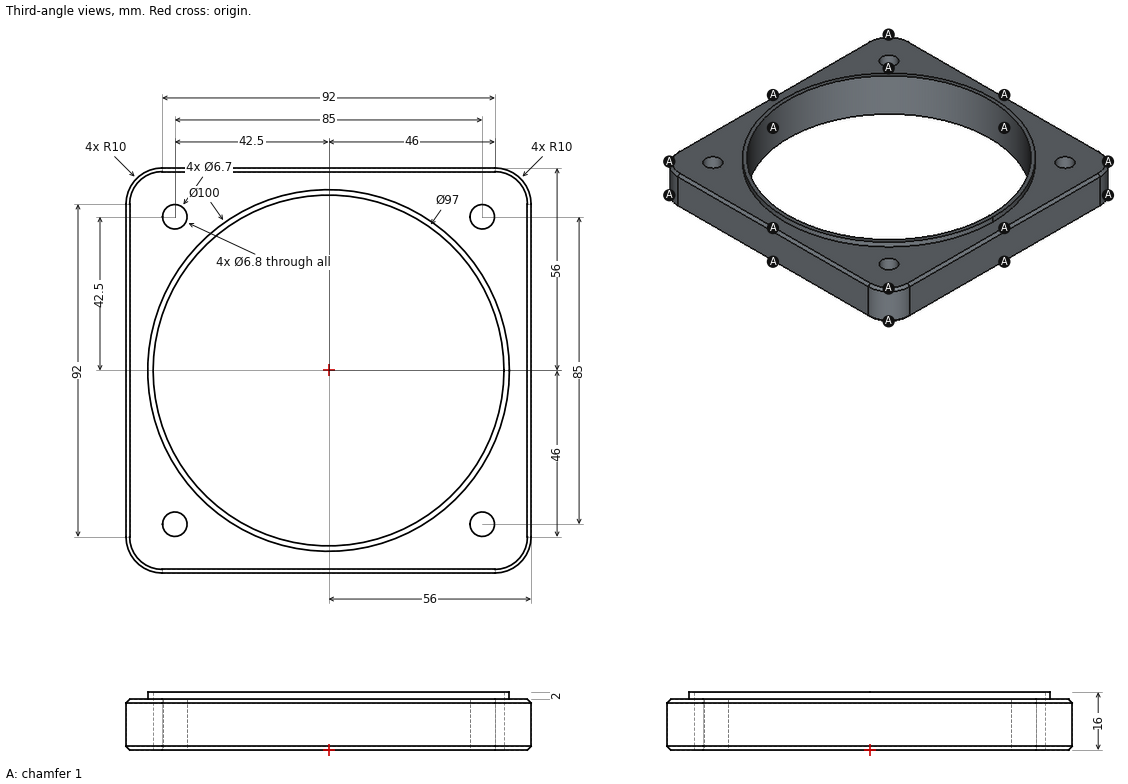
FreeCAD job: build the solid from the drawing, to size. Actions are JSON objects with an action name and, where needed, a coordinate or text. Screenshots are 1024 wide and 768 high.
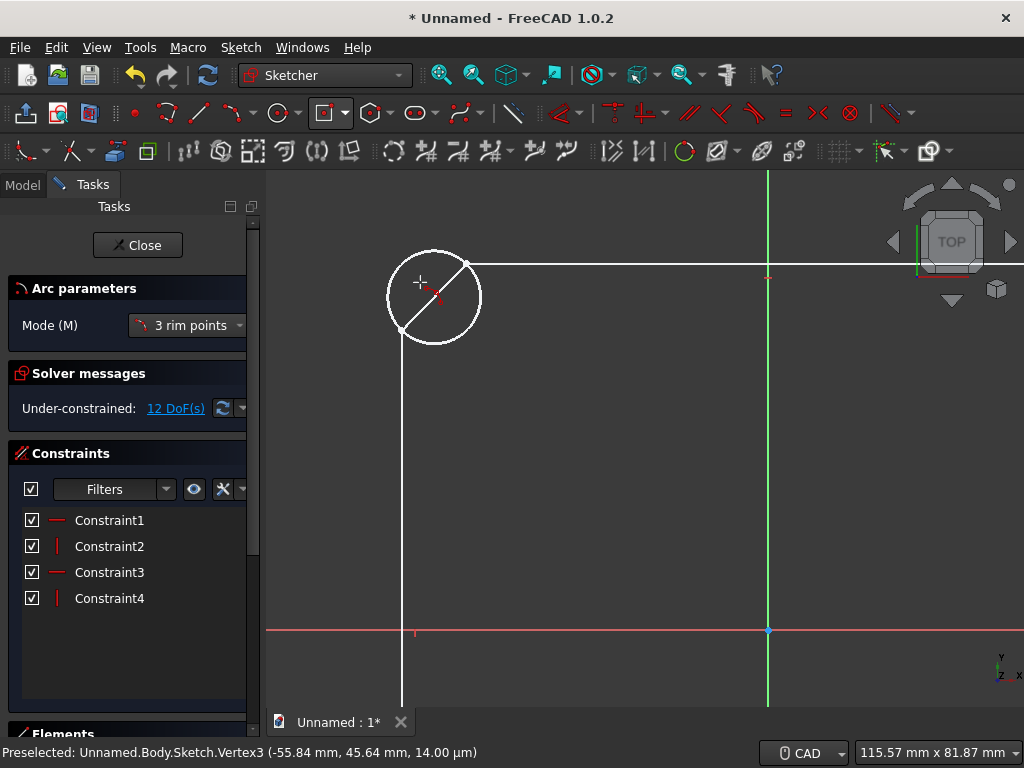
{"action": "left_click", "coordinate": [420, 282]}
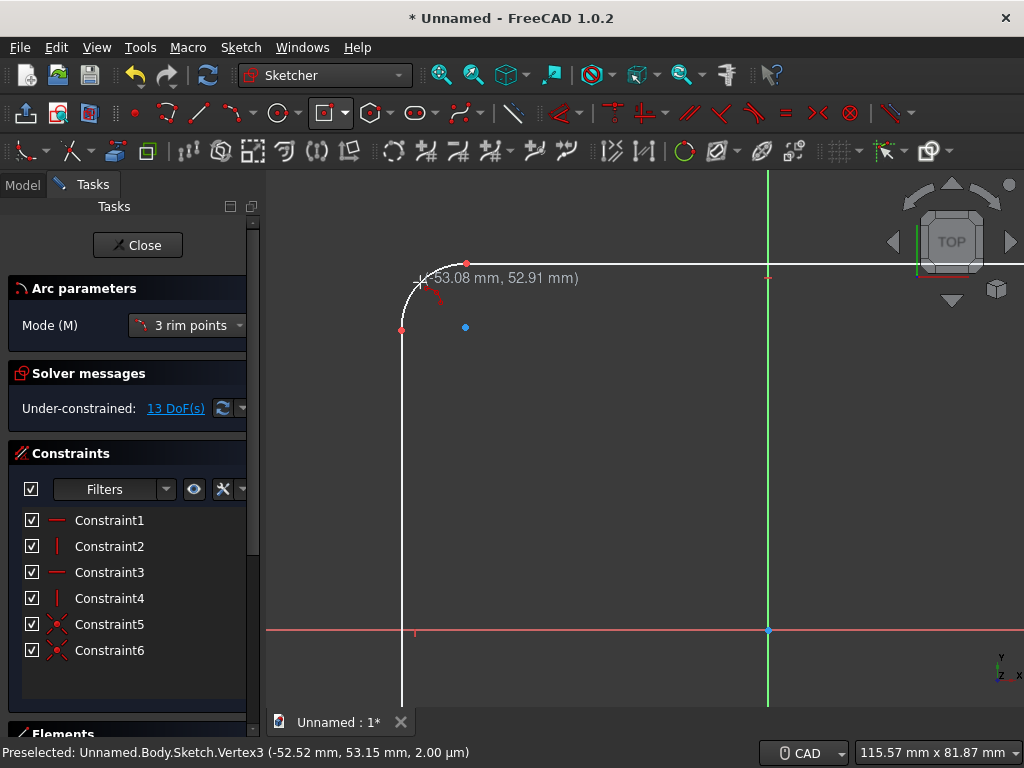
{"action": "scroll", "coordinate": [420, 282], "scroll_direction": "down", "scroll_amount": 4}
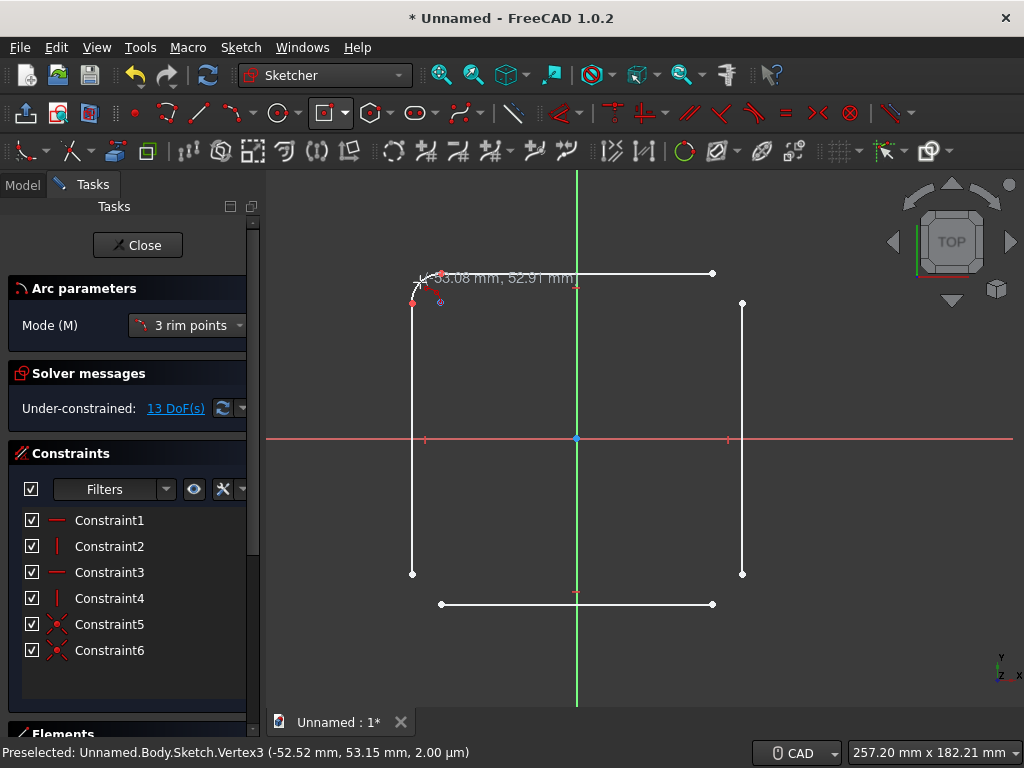
{"action": "left_click", "coordinate": [412, 575]}
{"action": "left_click", "coordinate": [441, 605]}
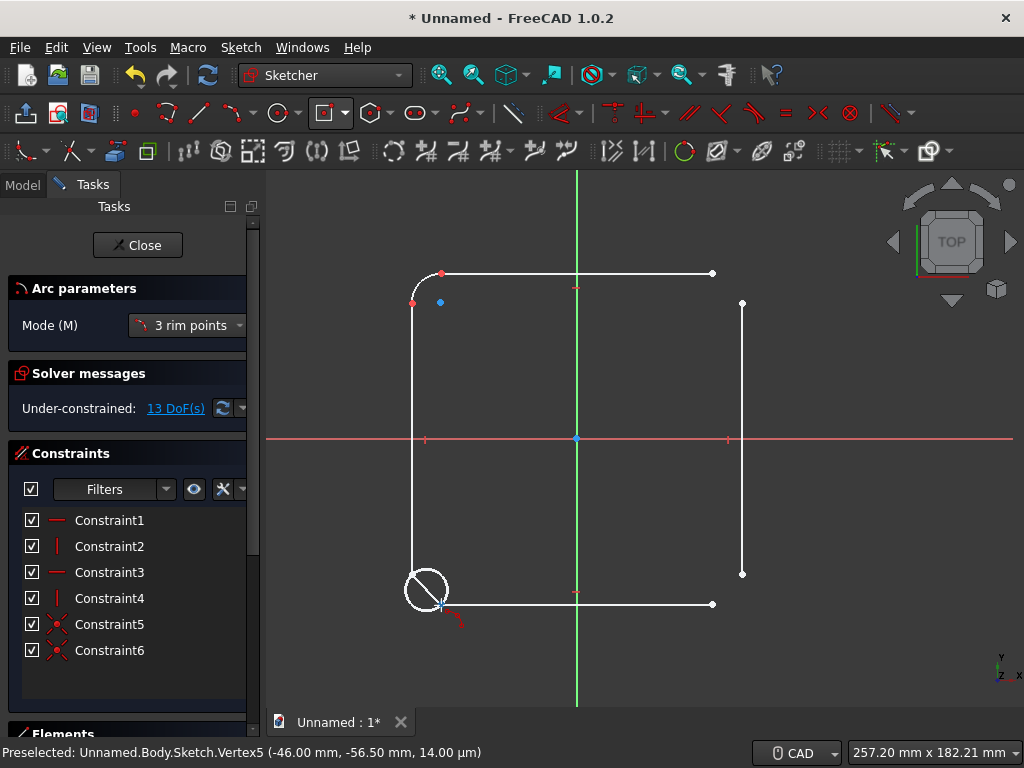
{"action": "scroll", "coordinate": [420, 595], "scroll_direction": "up", "scroll_amount": 4}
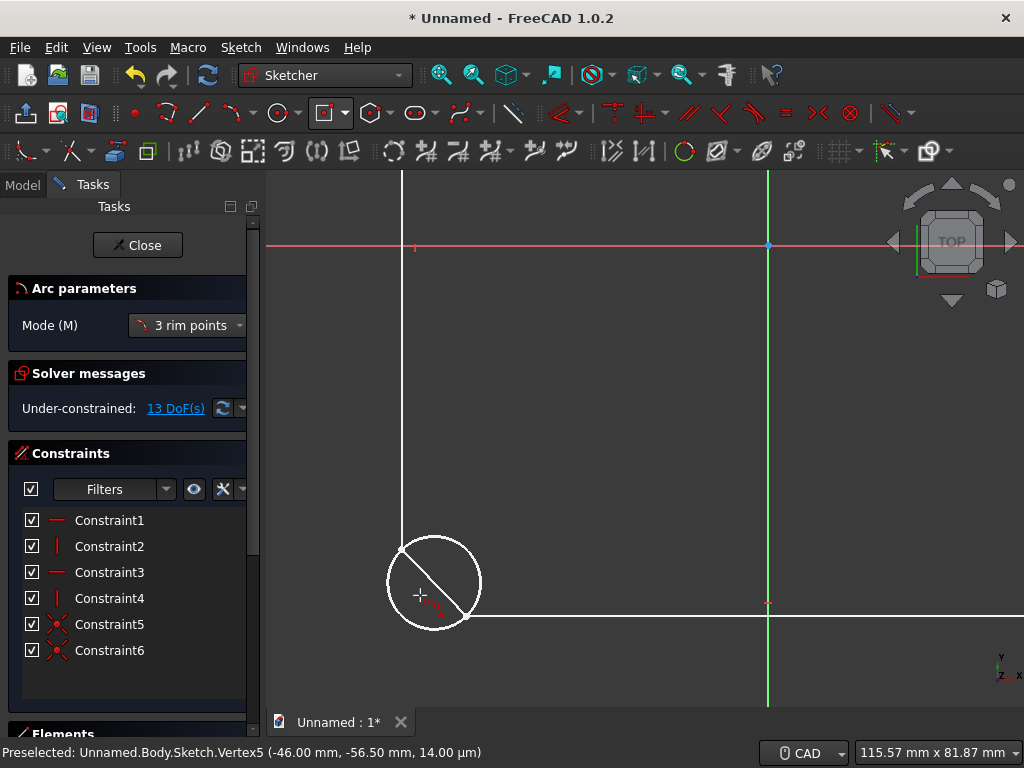
{"action": "left_click", "coordinate": [420, 594]}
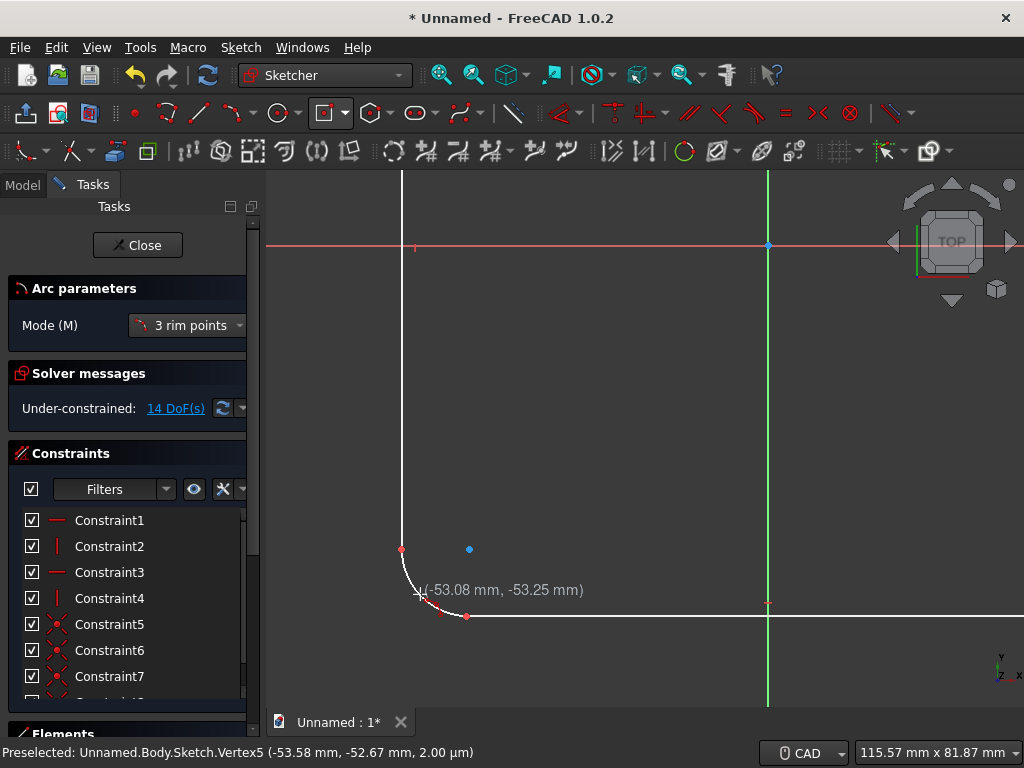
{"action": "scroll", "coordinate": [420, 596], "scroll_direction": "down", "scroll_amount": 4}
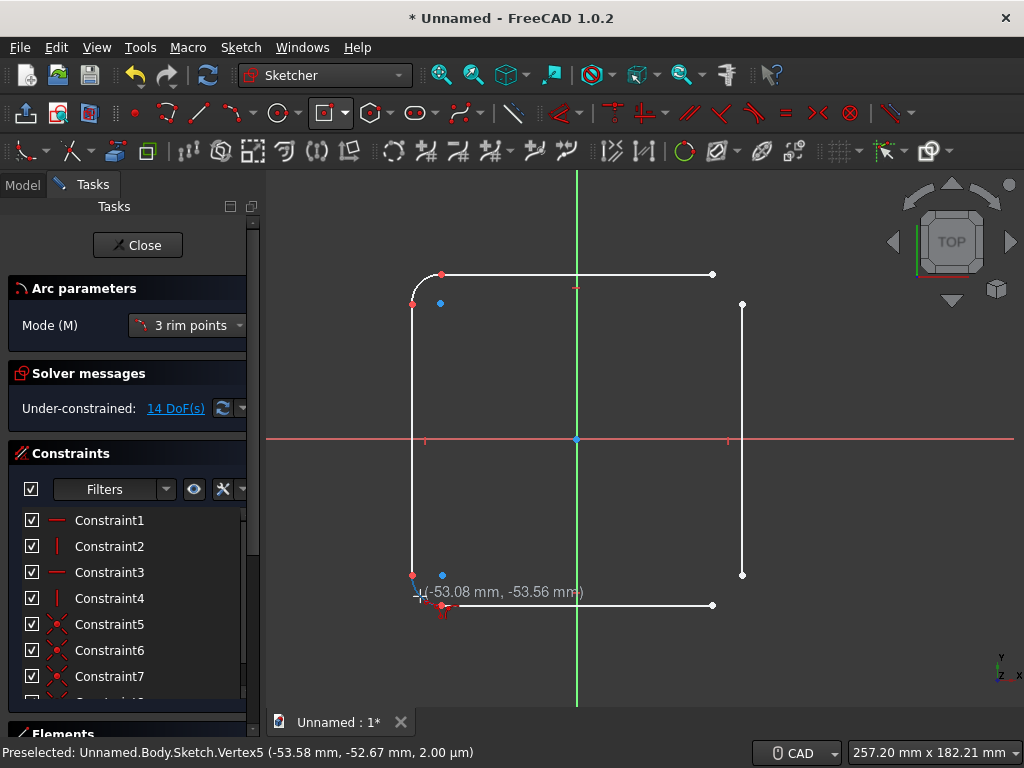
{"action": "left_click", "coordinate": [712, 606]}
{"action": "left_click", "coordinate": [742, 576]}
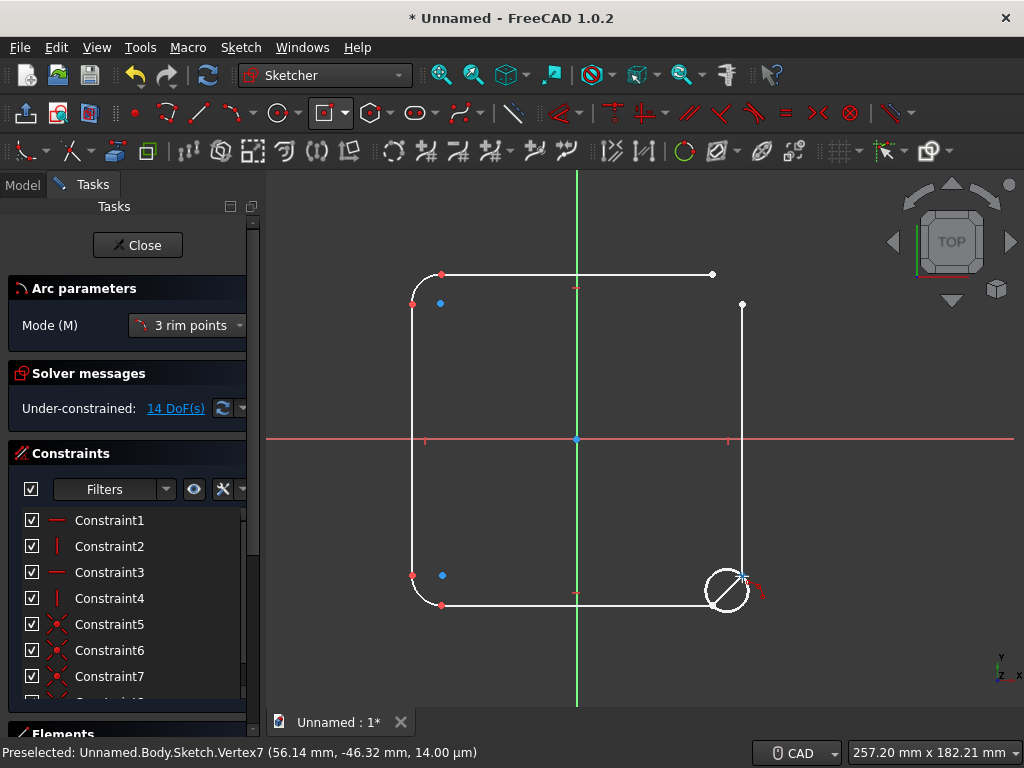
{"action": "scroll", "coordinate": [733, 595], "scroll_direction": "up", "scroll_amount": 4}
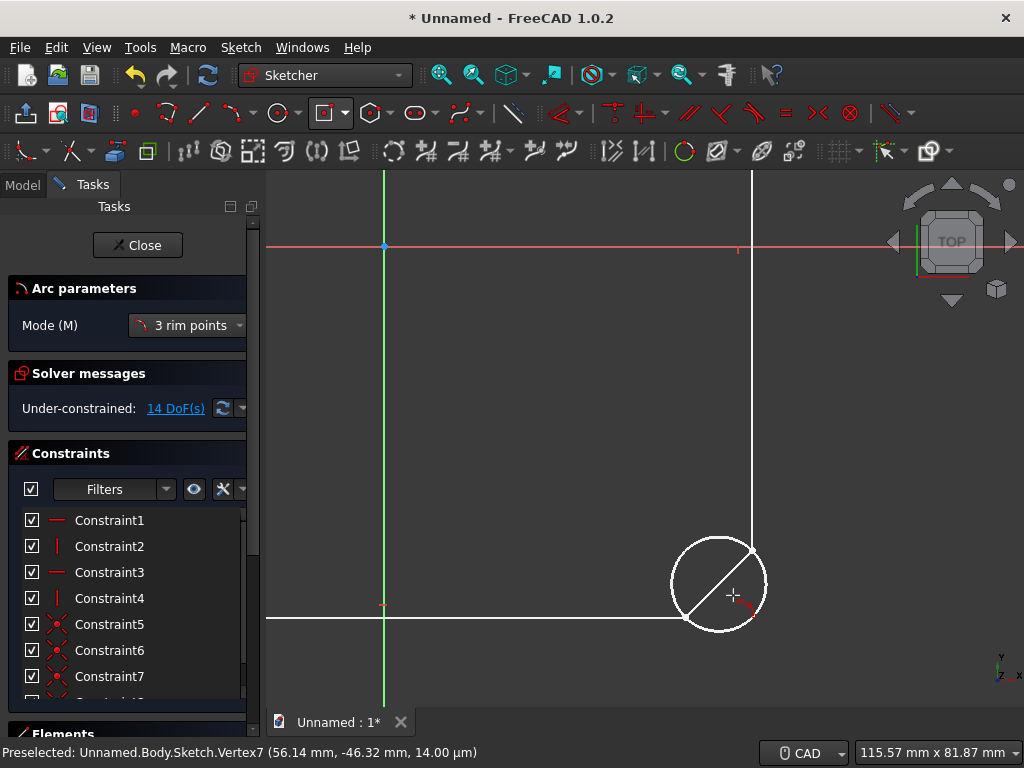
{"action": "left_click", "coordinate": [732, 595]}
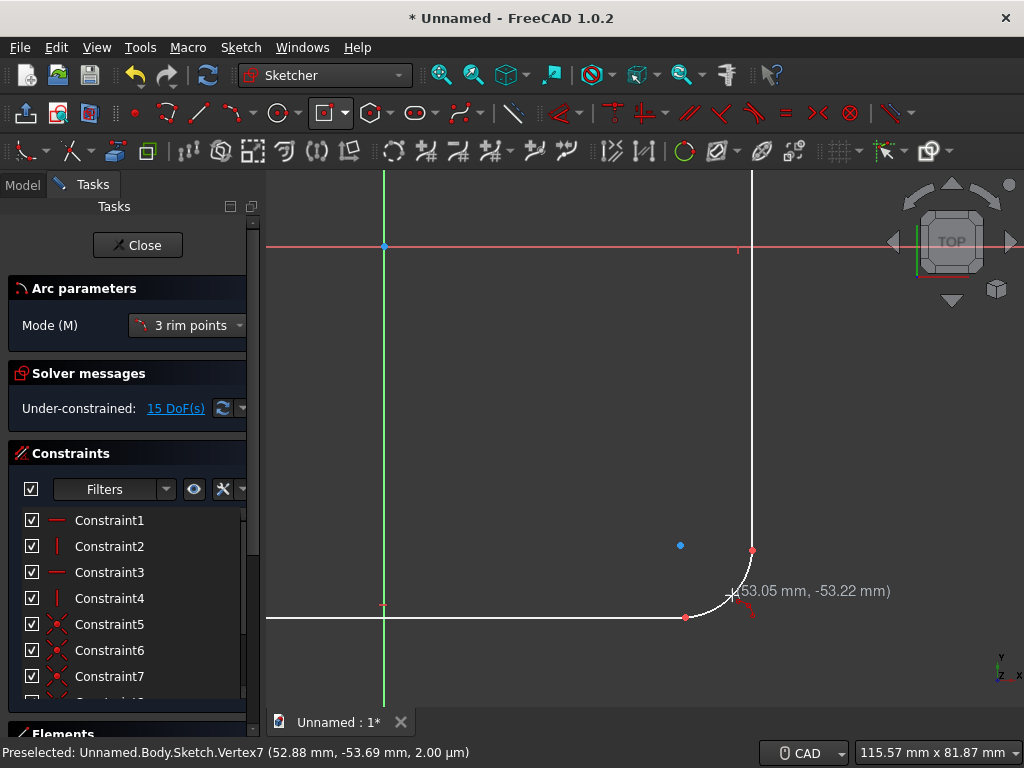
{"action": "scroll", "coordinate": [734, 595], "scroll_direction": "down", "scroll_amount": 4}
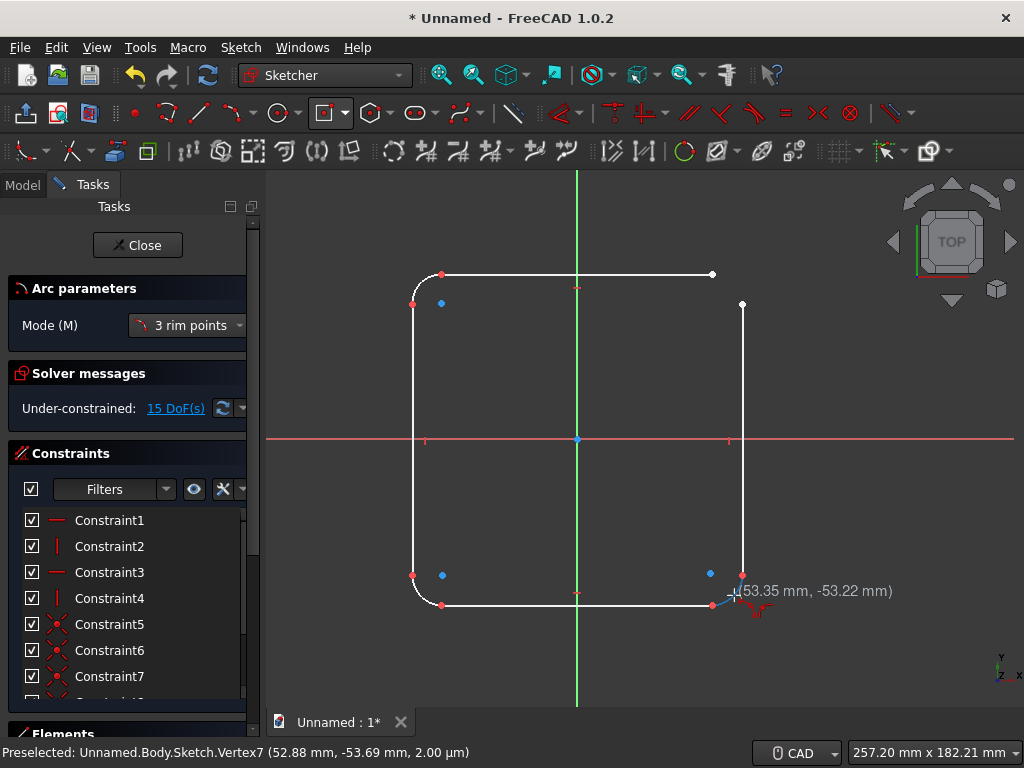
{"action": "left_click", "coordinate": [743, 305]}
{"action": "left_click", "coordinate": [713, 275]}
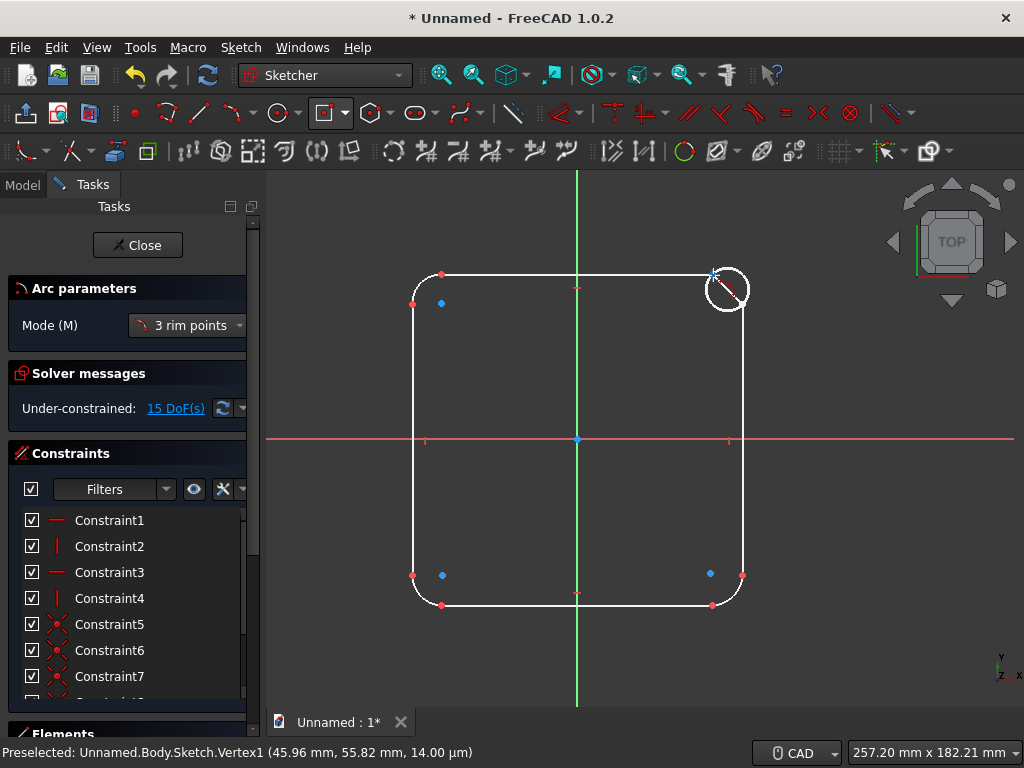
{"action": "scroll", "coordinate": [734, 283], "scroll_direction": "up", "scroll_amount": 4}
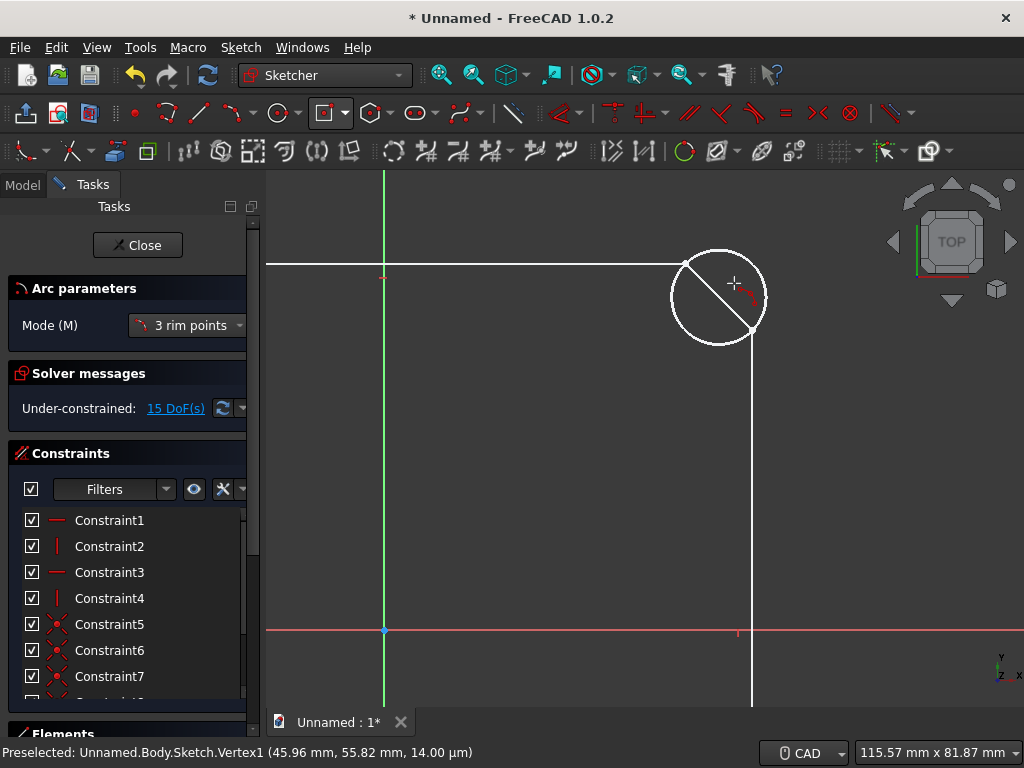
{"action": "left_click", "coordinate": [732, 282]}